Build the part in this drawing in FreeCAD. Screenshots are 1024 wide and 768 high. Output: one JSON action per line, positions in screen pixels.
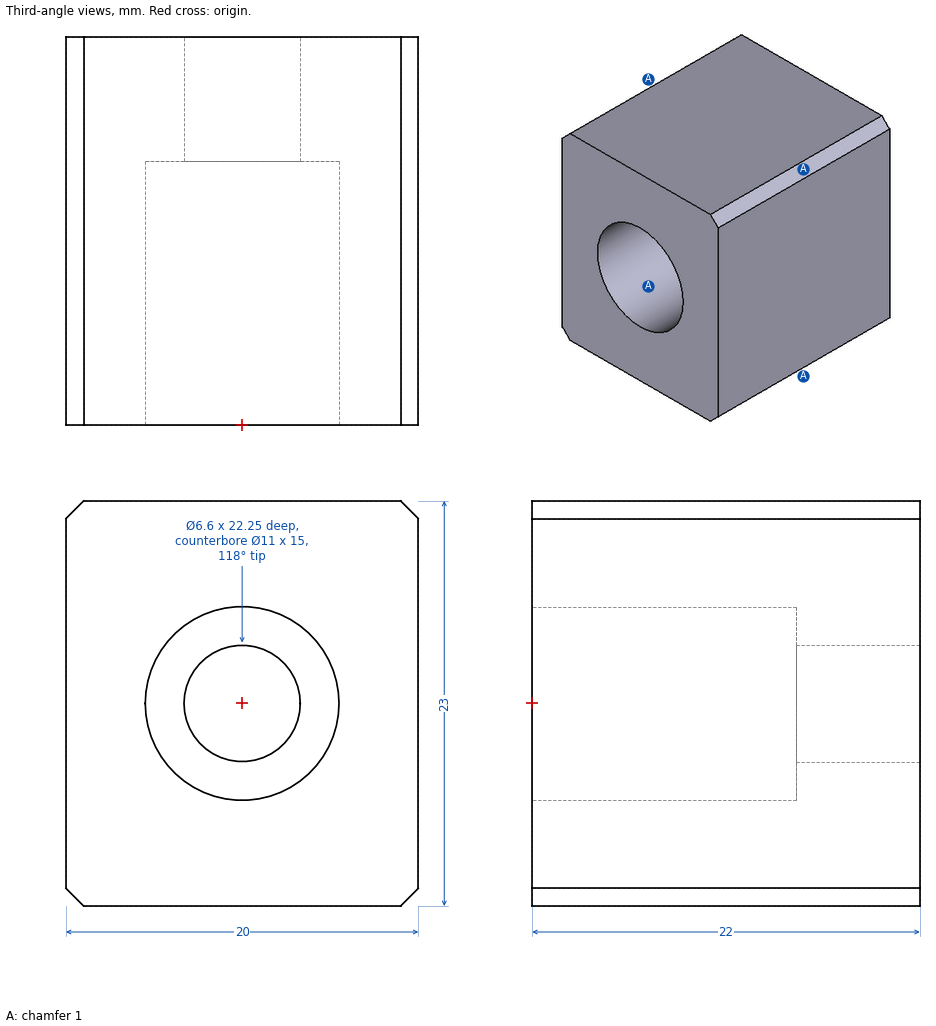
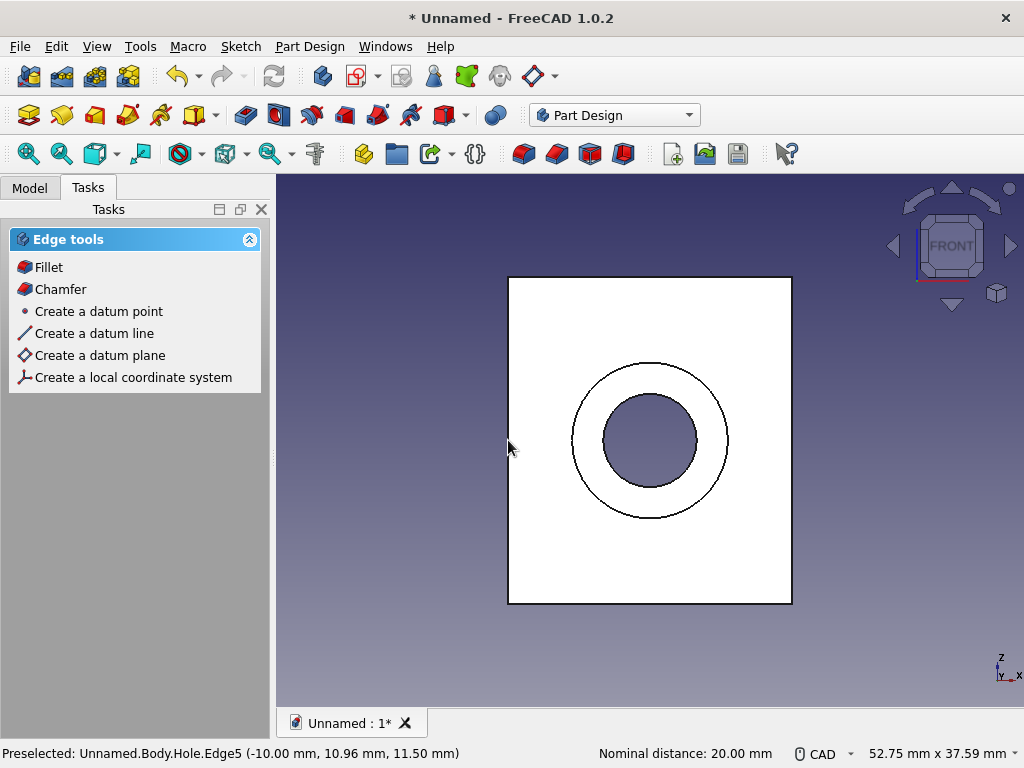
{"action": "key", "text": "3"}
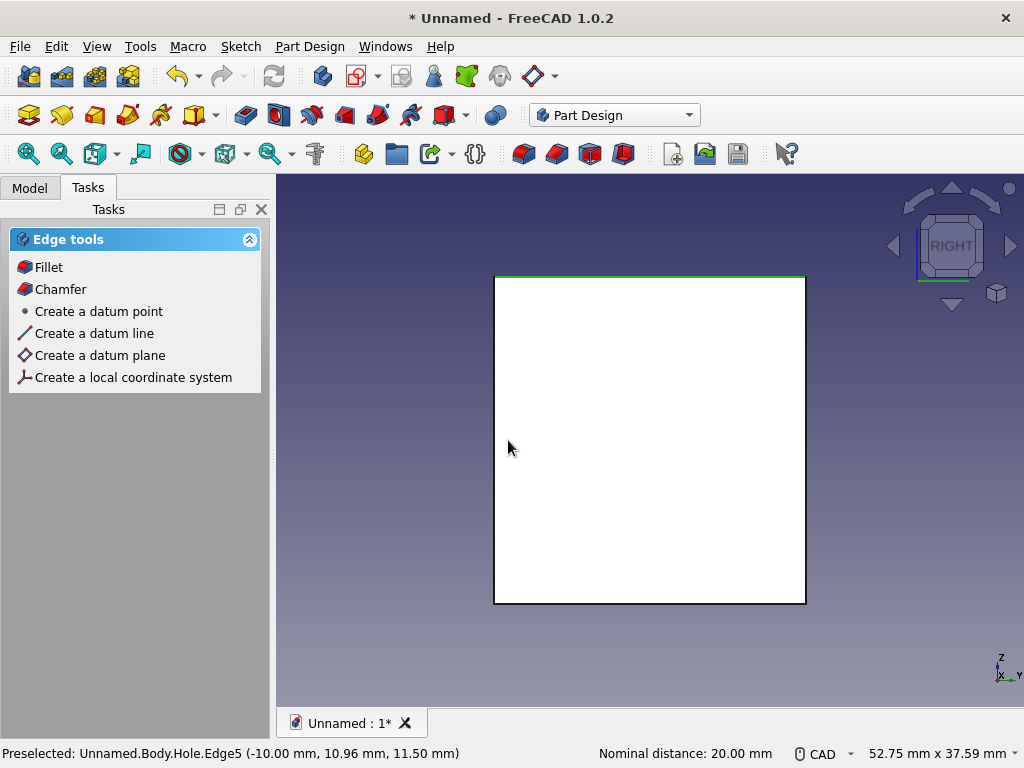
{"action": "left_click", "coordinate": [650, 603], "text": "ctrl"}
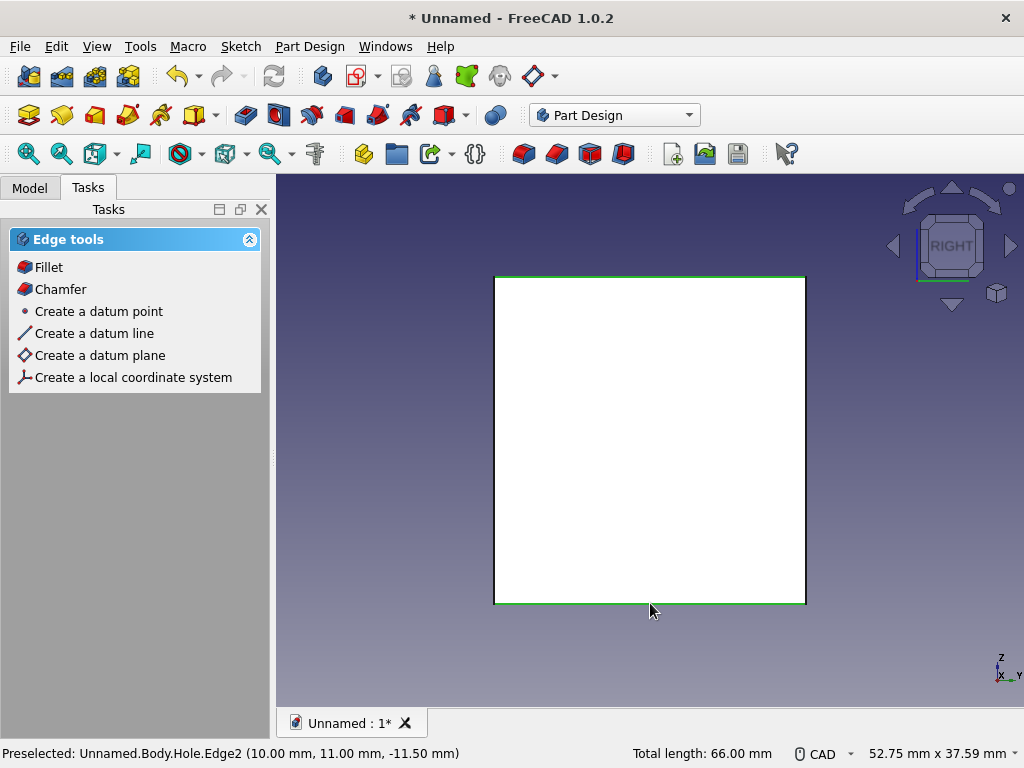
{"action": "key", "text": "5"}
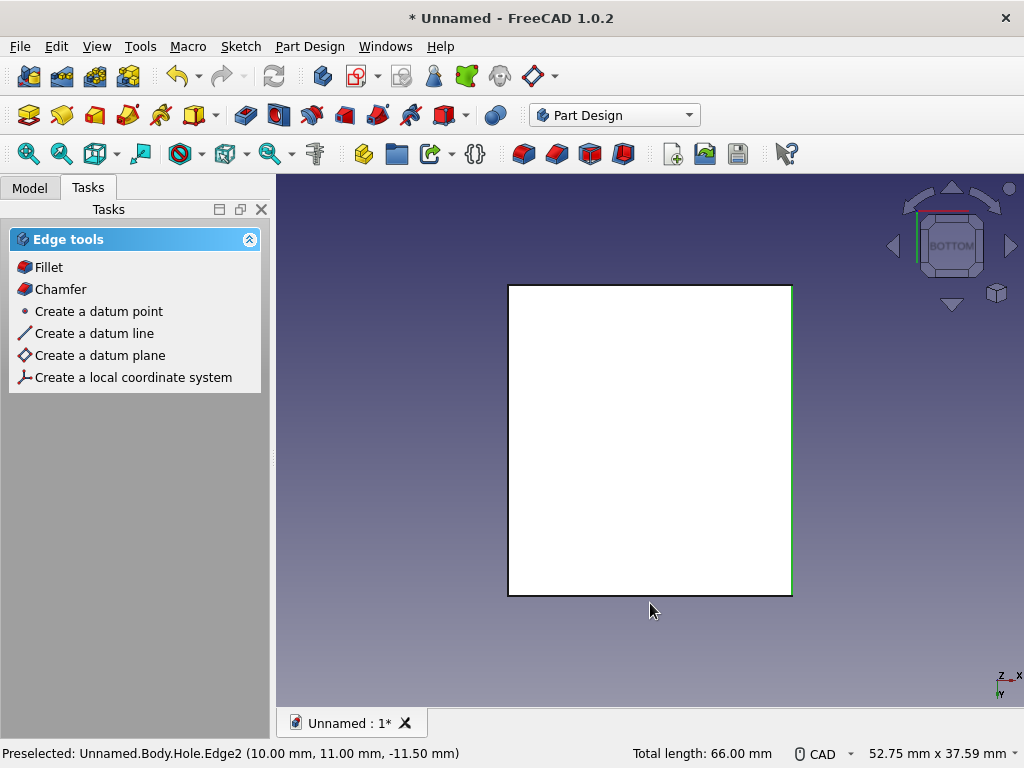
{"action": "left_click", "coordinate": [508, 440], "text": "ctrl"}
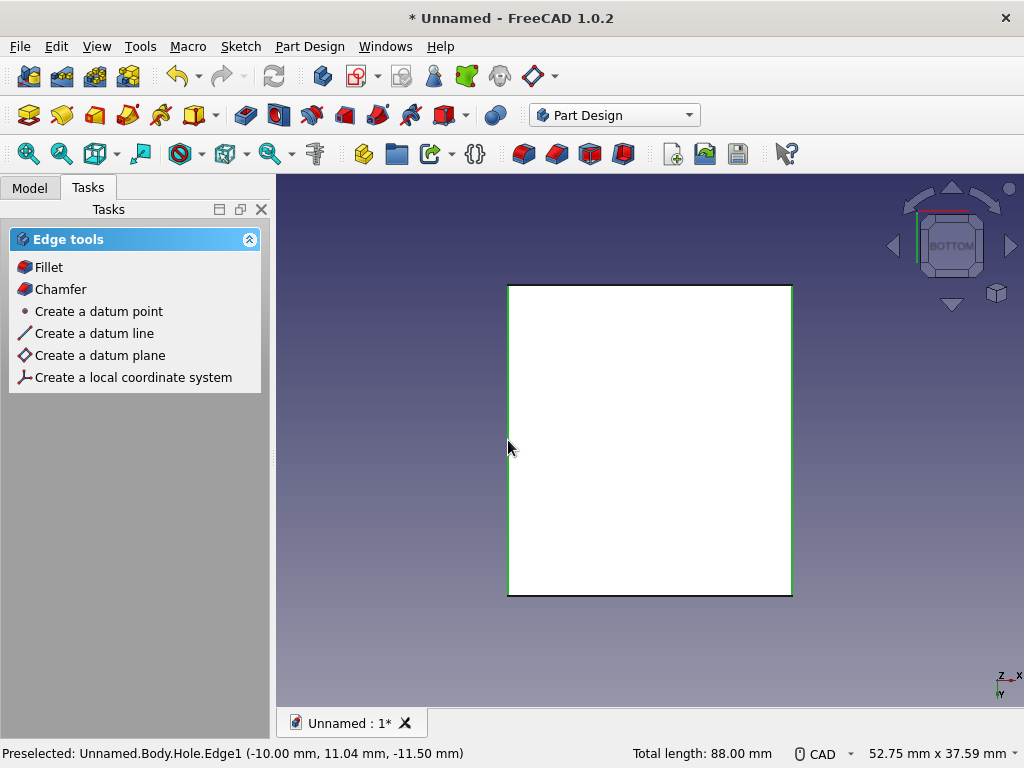
{"action": "left_click", "coordinate": [557, 154]}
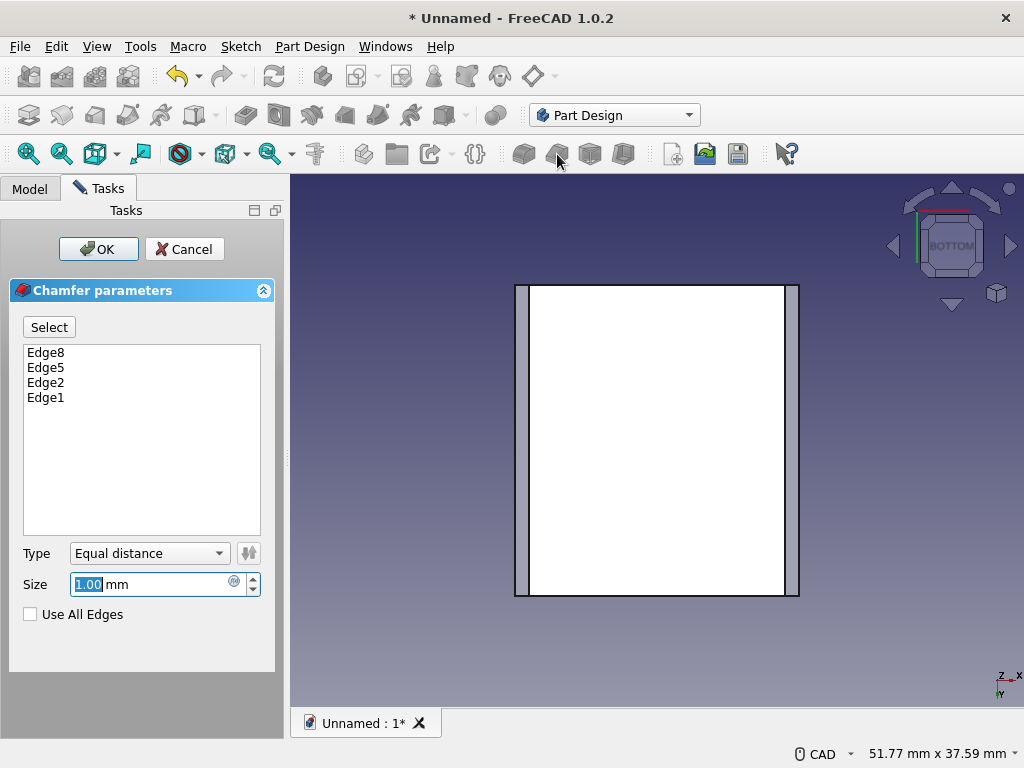
{"action": "type", "text": "1"}
{"action": "key", "text": "Tab"}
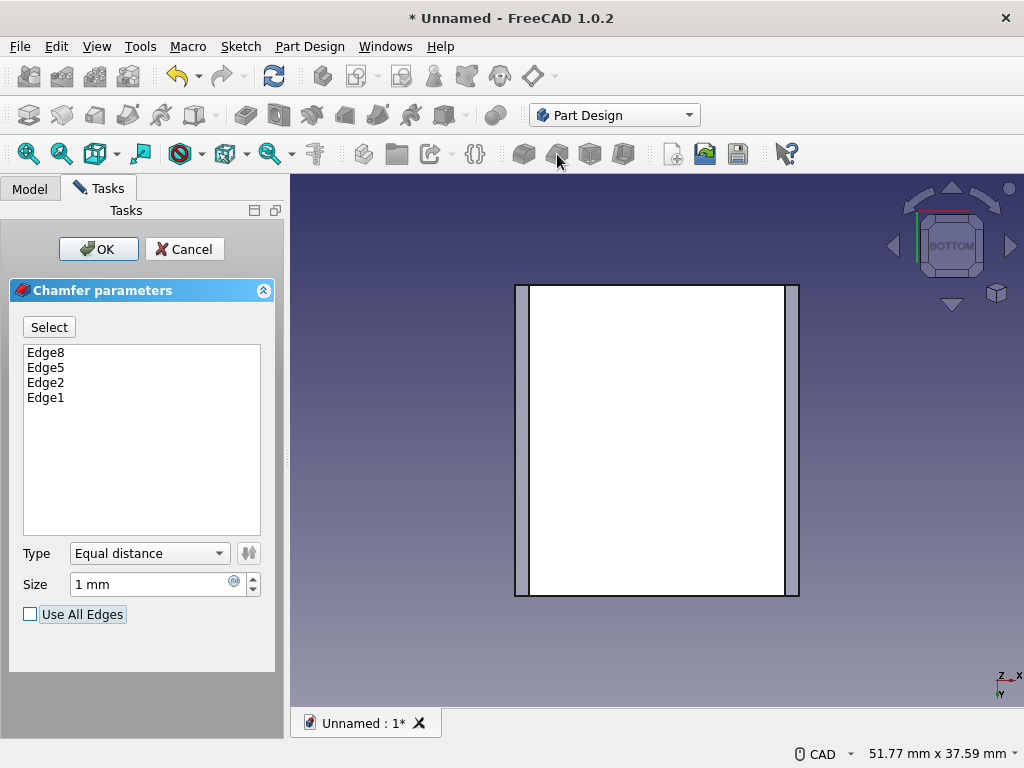
{"action": "left_click", "coordinate": [99, 249]}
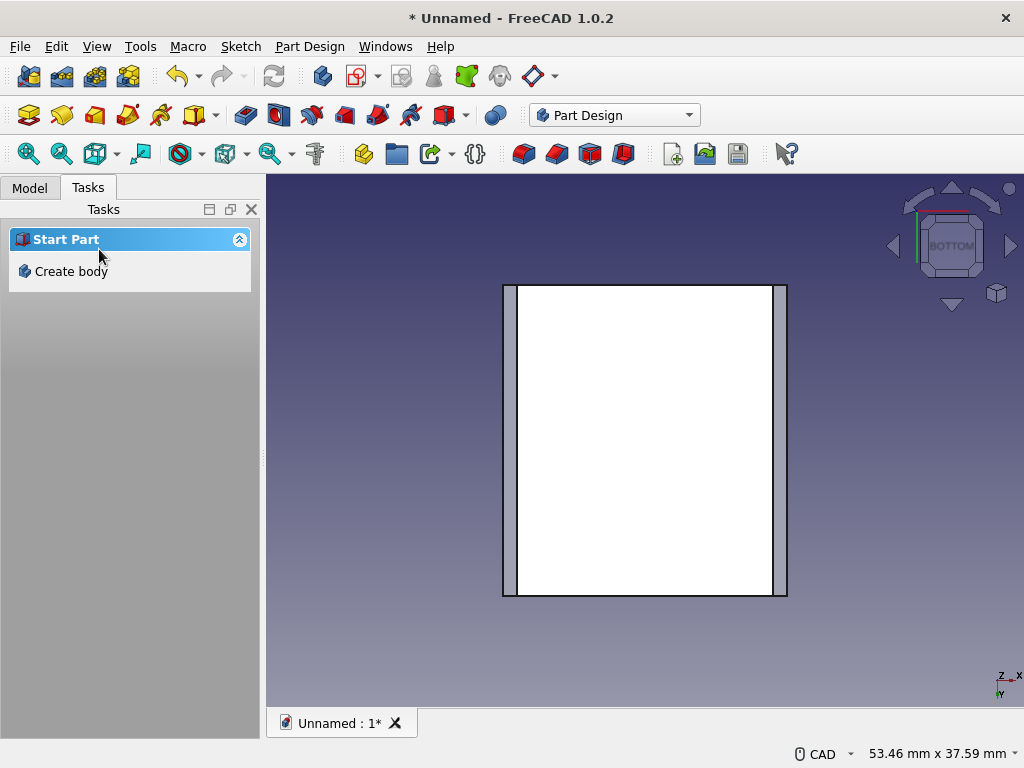
{"action": "key", "text": "0"}